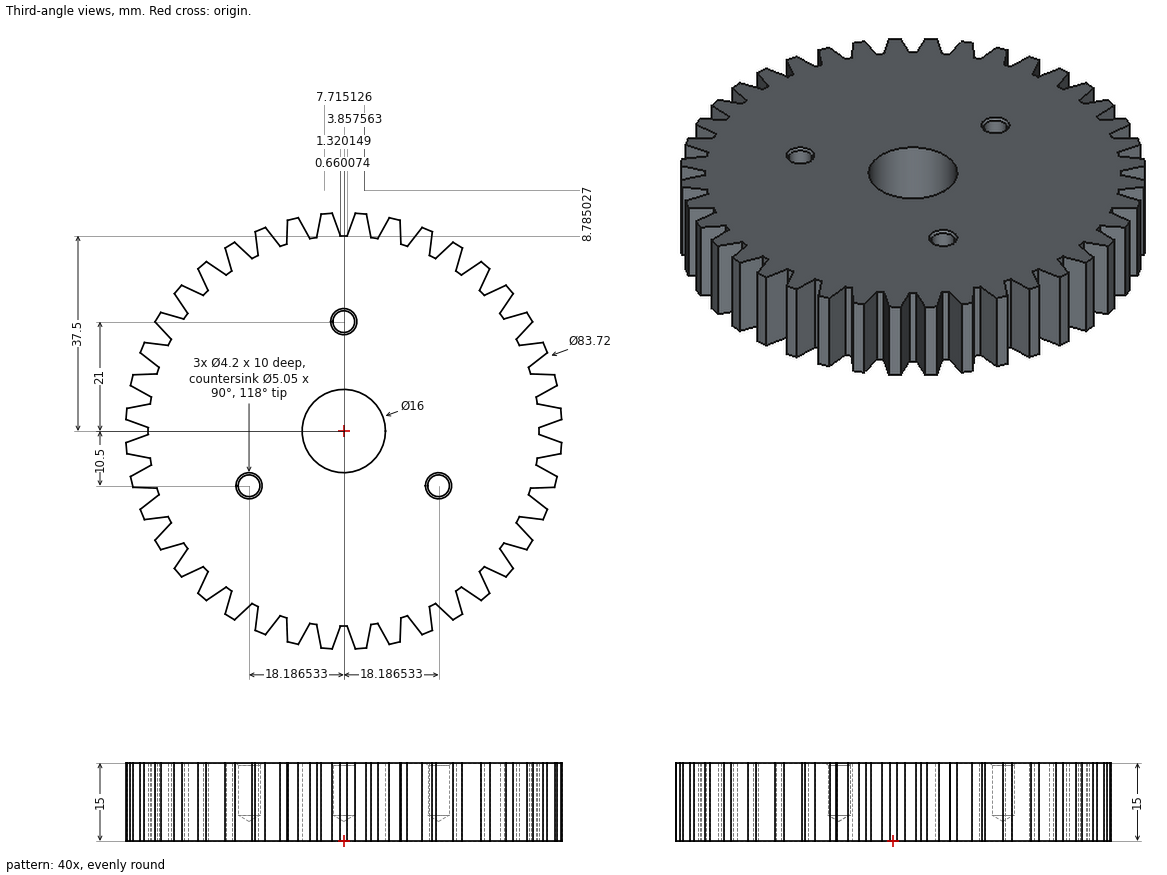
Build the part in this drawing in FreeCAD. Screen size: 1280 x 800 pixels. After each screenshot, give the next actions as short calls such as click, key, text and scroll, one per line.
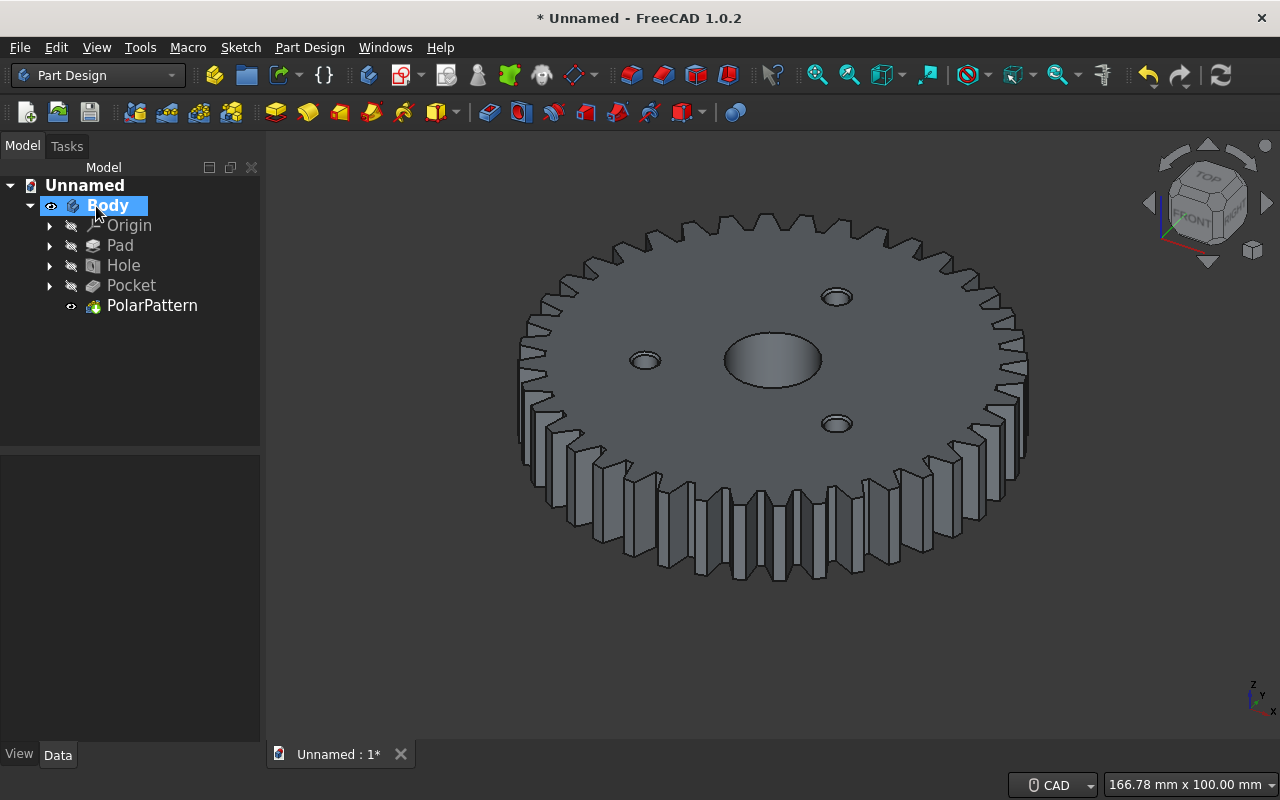
key(0)